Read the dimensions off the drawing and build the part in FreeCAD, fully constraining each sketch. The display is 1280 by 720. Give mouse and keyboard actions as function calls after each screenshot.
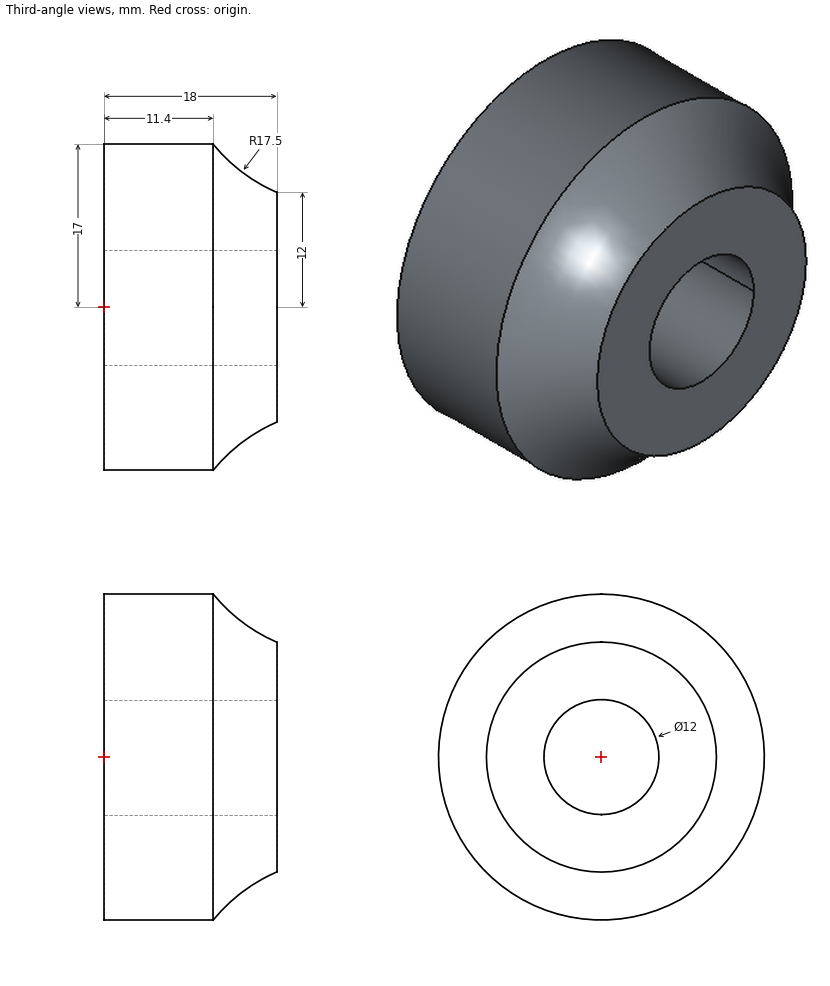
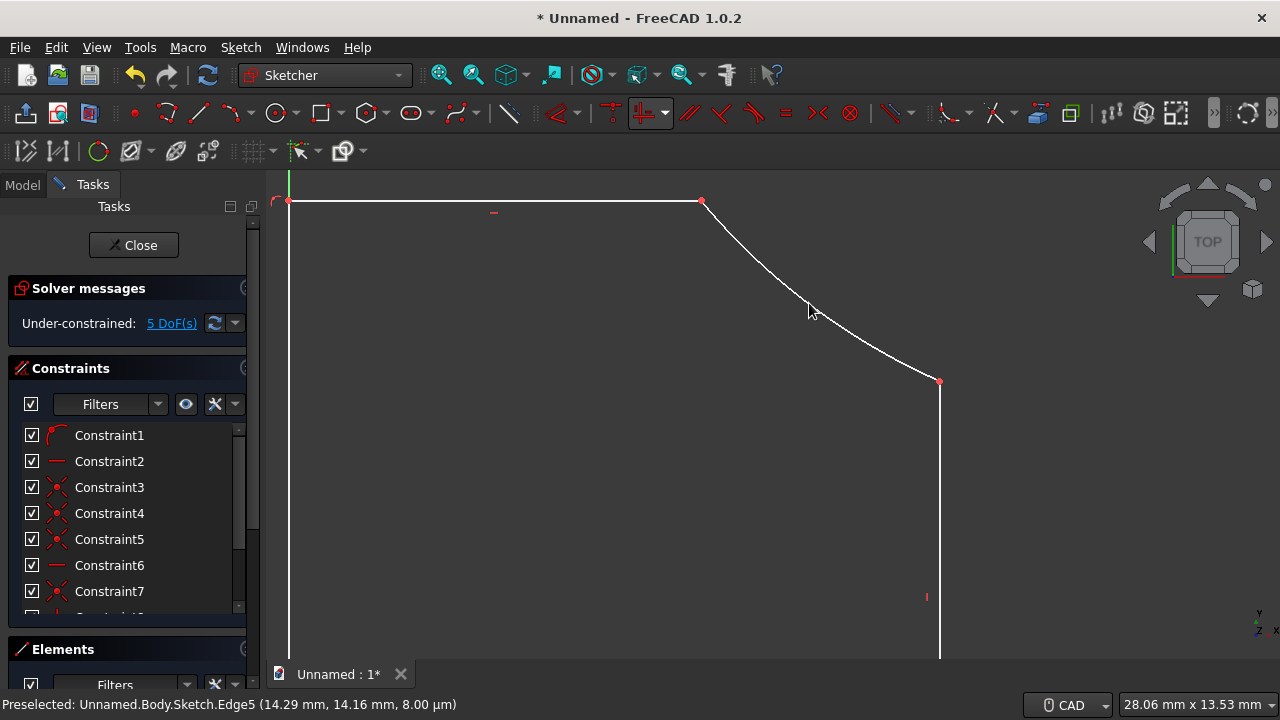
click(556, 114)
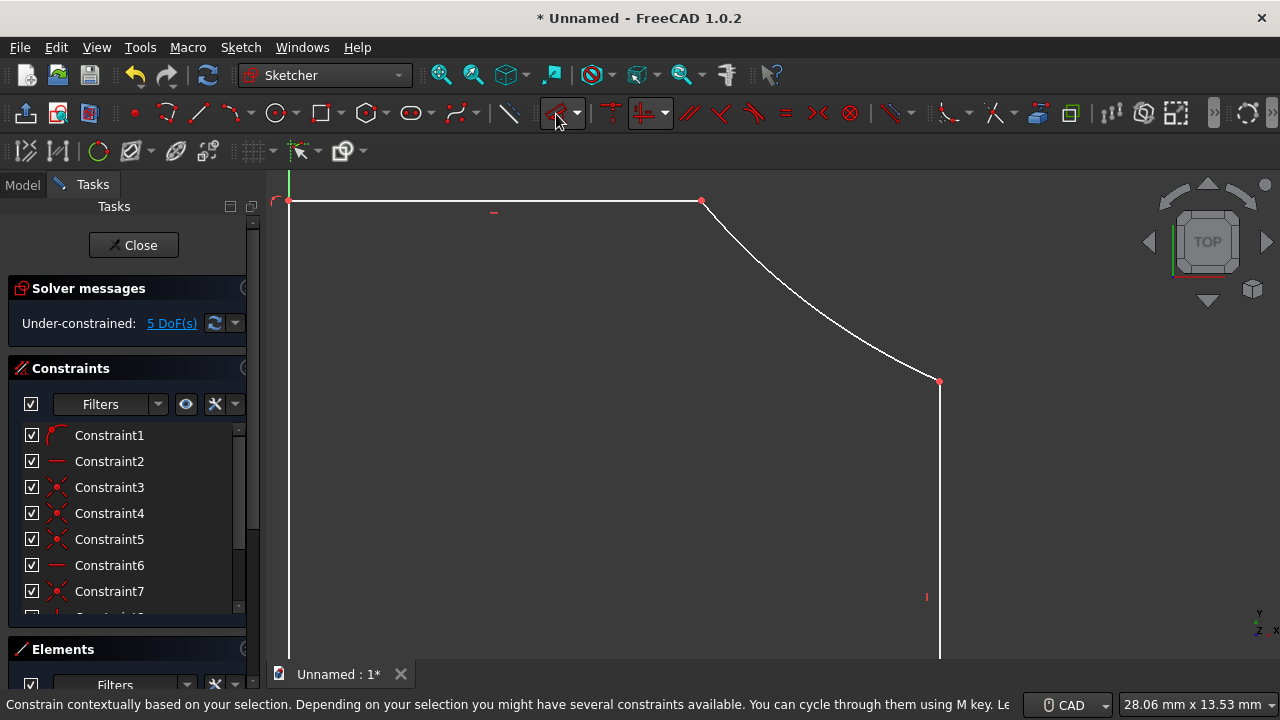
click(764, 266)
click(742, 290)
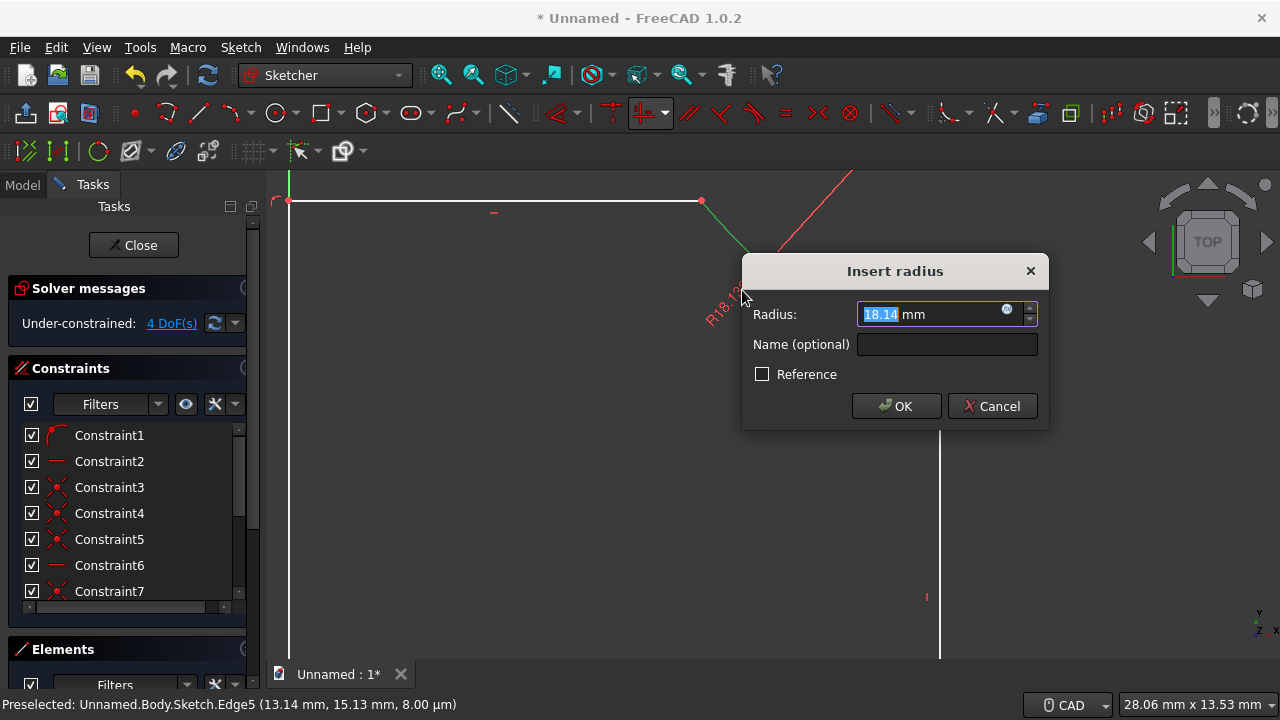
text(17.5)
key(Return)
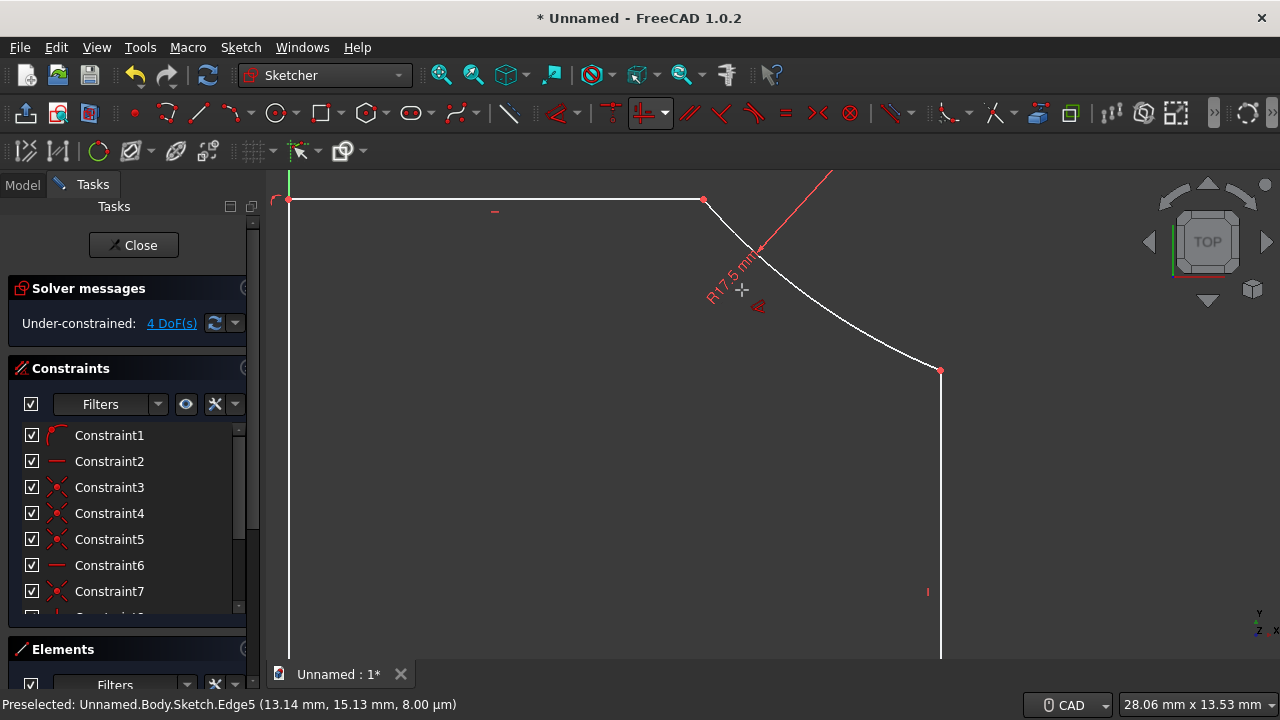
scroll(815, 304, down, 3)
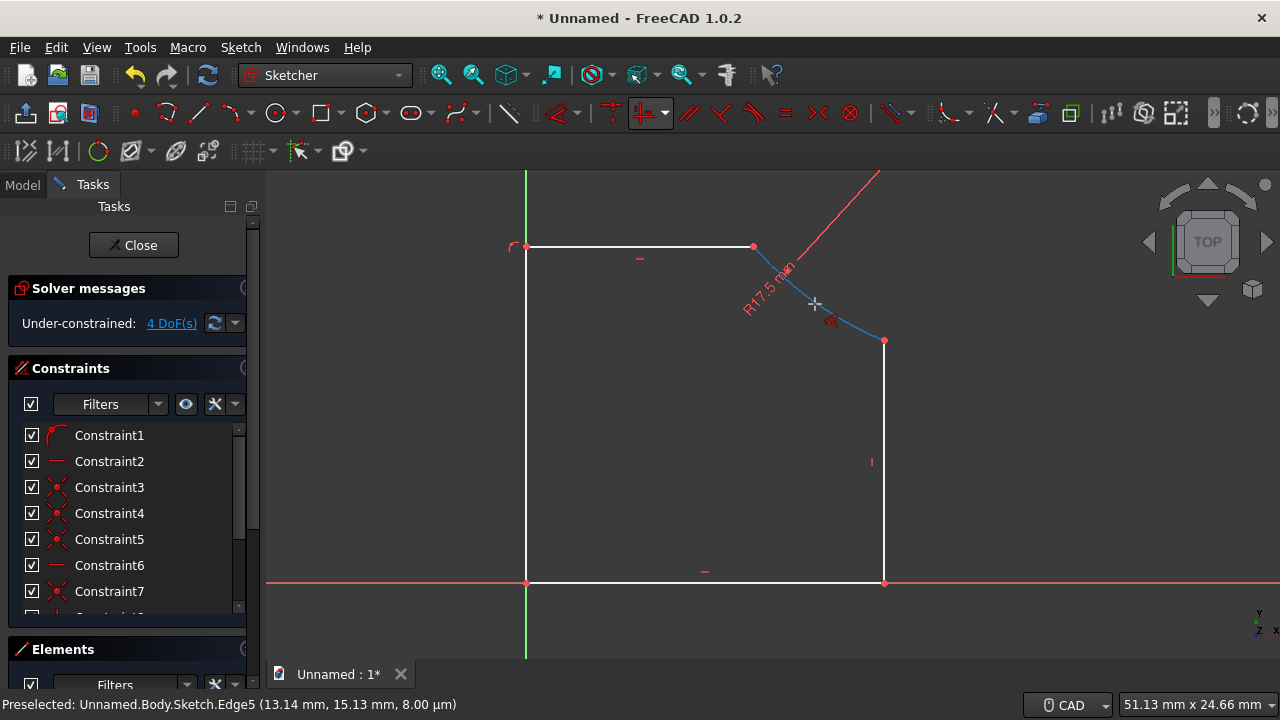
click(526, 348)
click(492, 415)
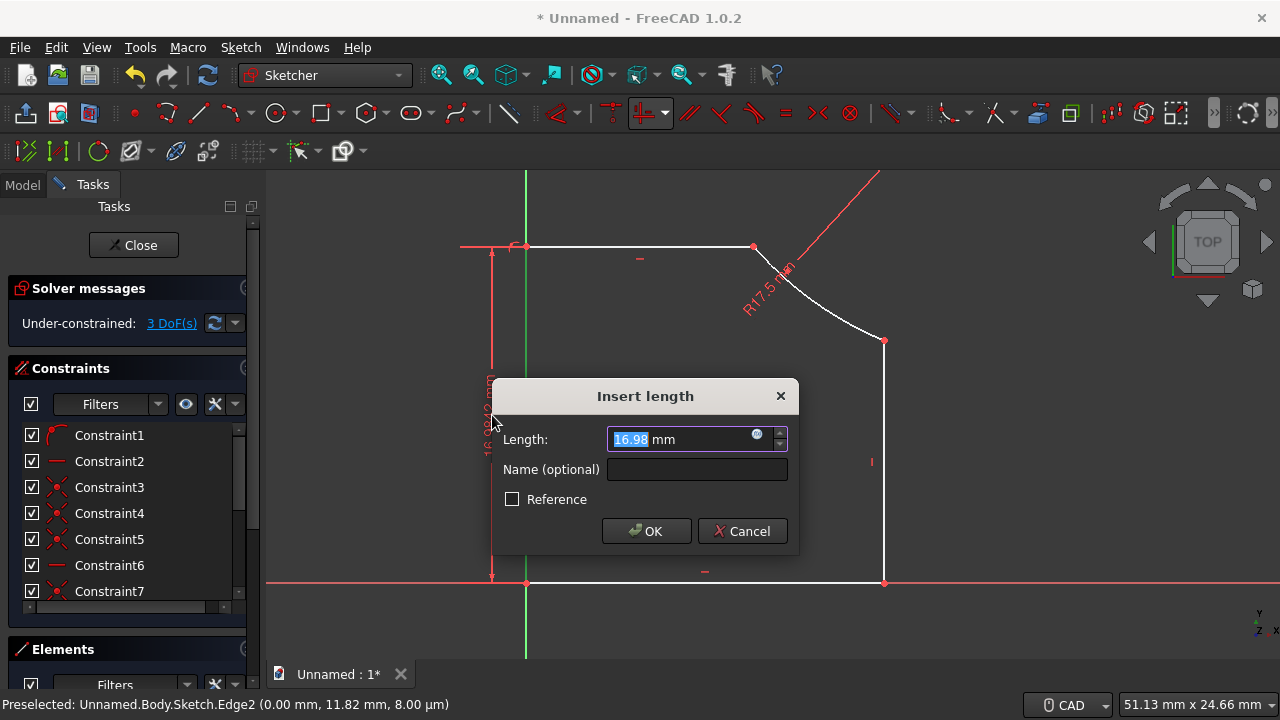
text(17)
key(Return)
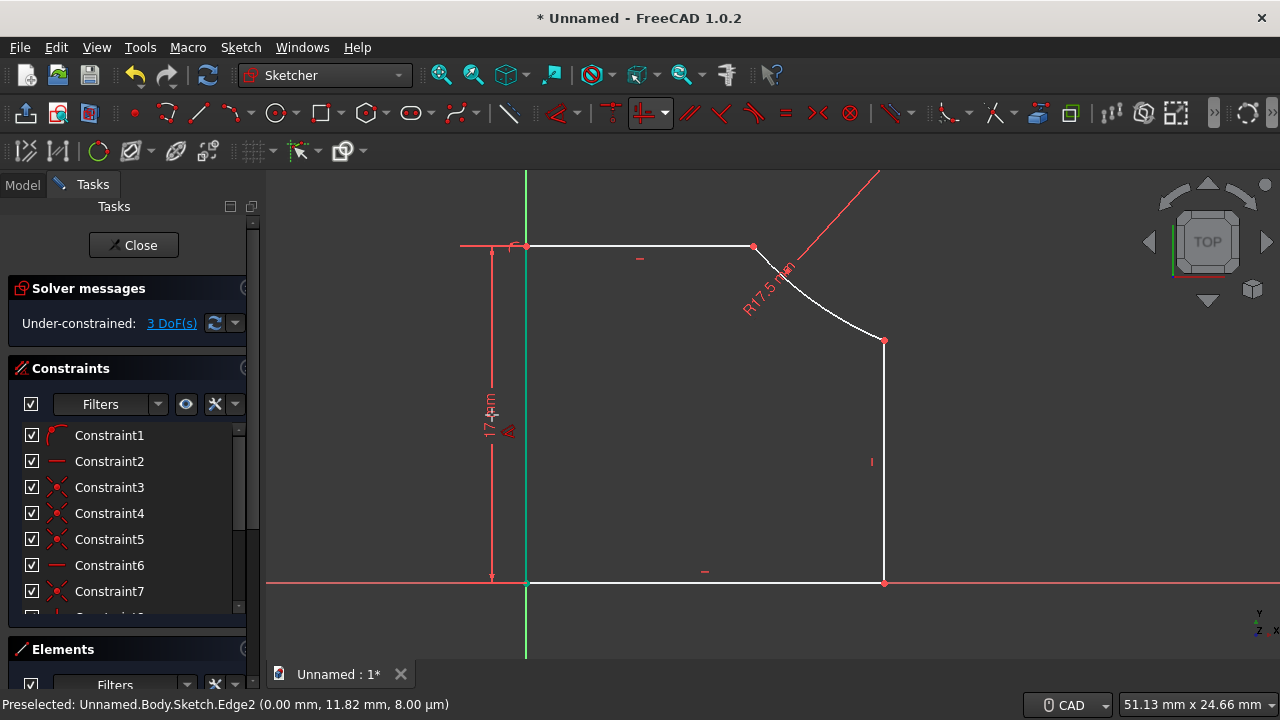
click(634, 583)
click(705, 617)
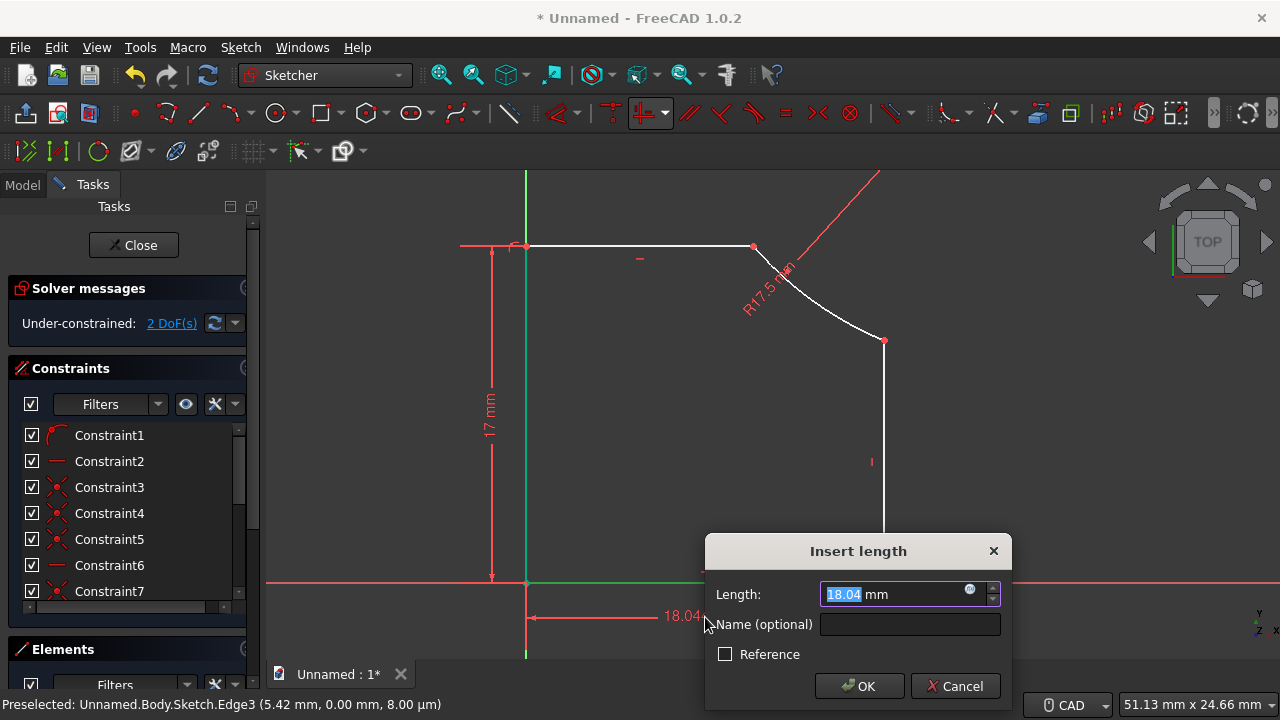
text(18)
key(Return)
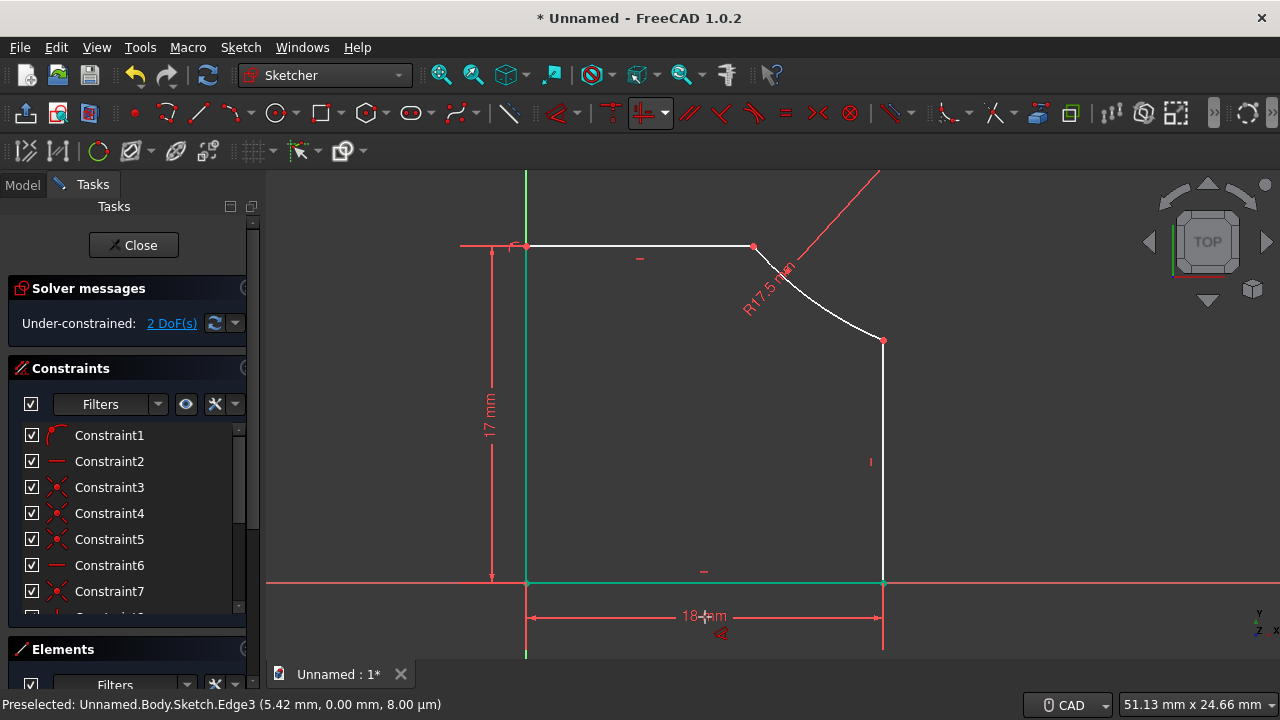
click(883, 510)
click(917, 462)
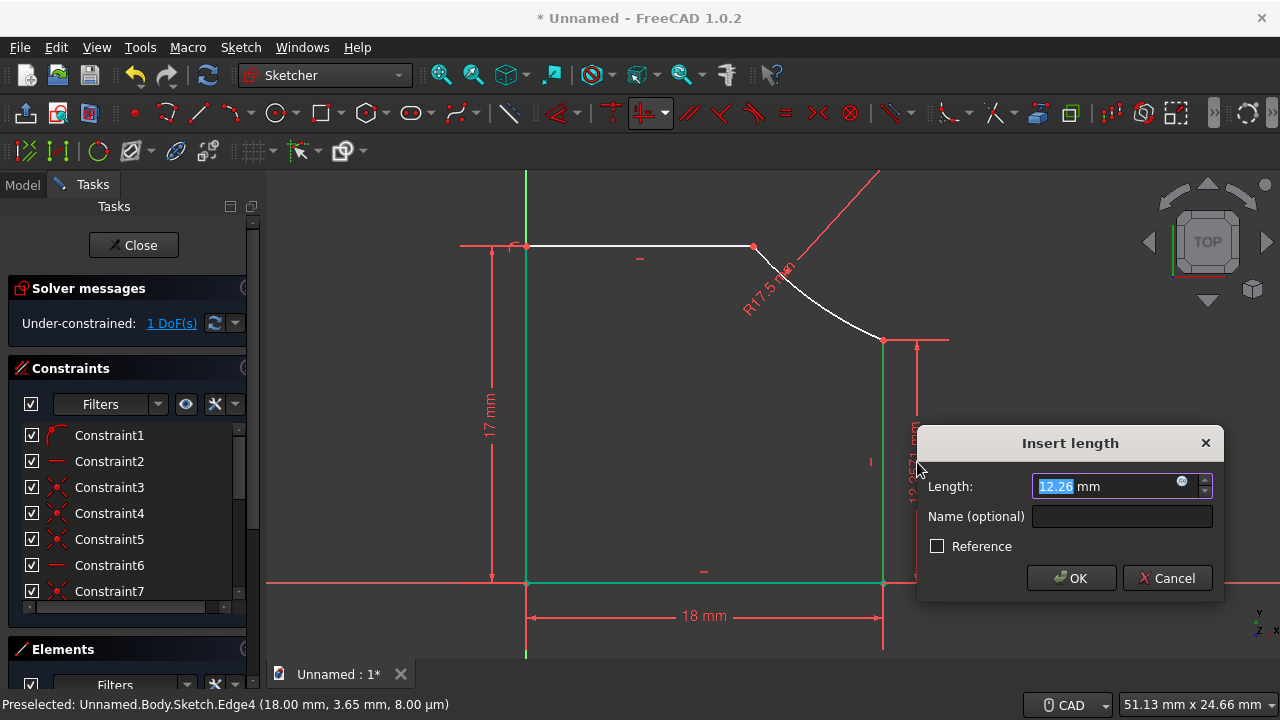
text(12)
key(Return)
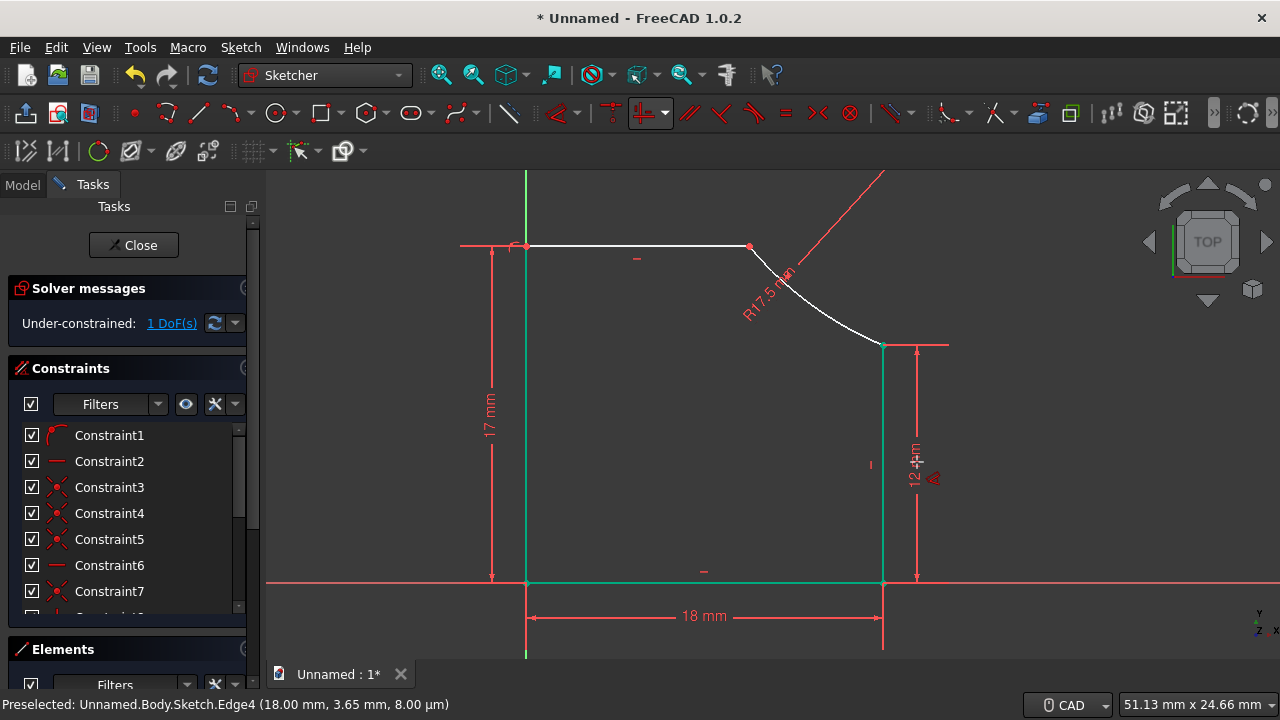
click(682, 246)
click(638, 212)